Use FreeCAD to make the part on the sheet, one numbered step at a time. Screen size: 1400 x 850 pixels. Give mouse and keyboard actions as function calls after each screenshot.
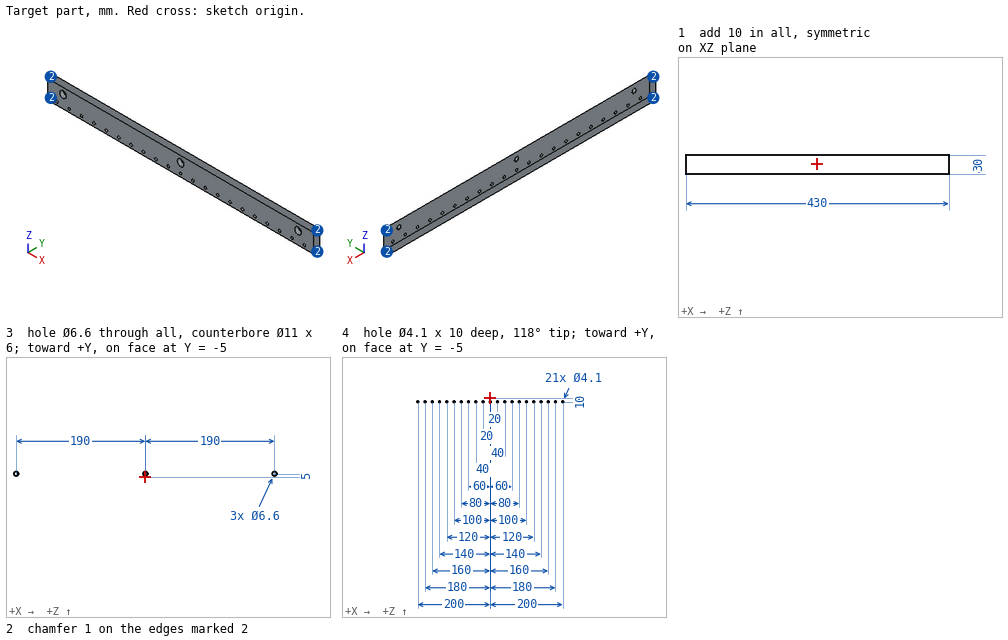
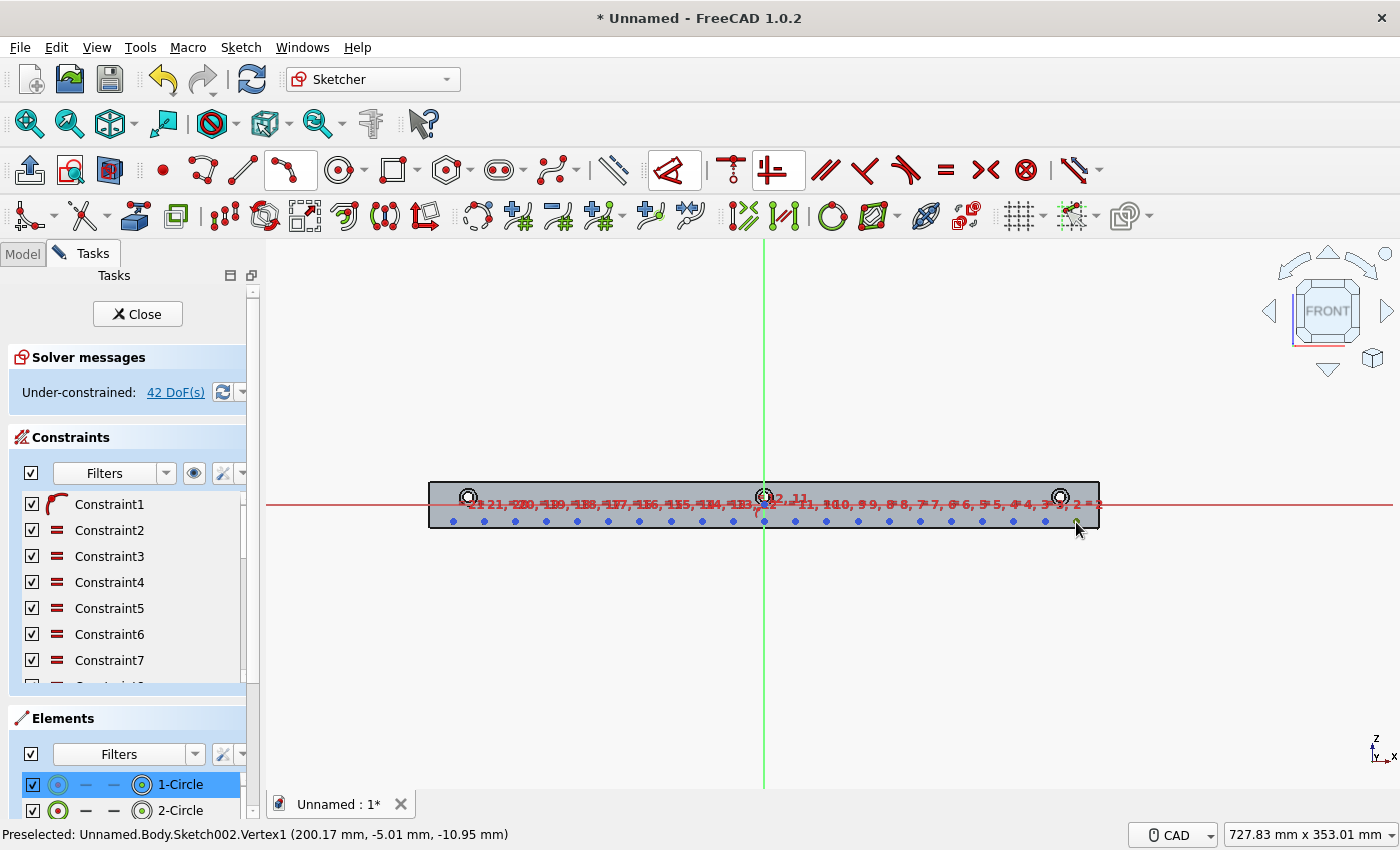
click(1045, 522)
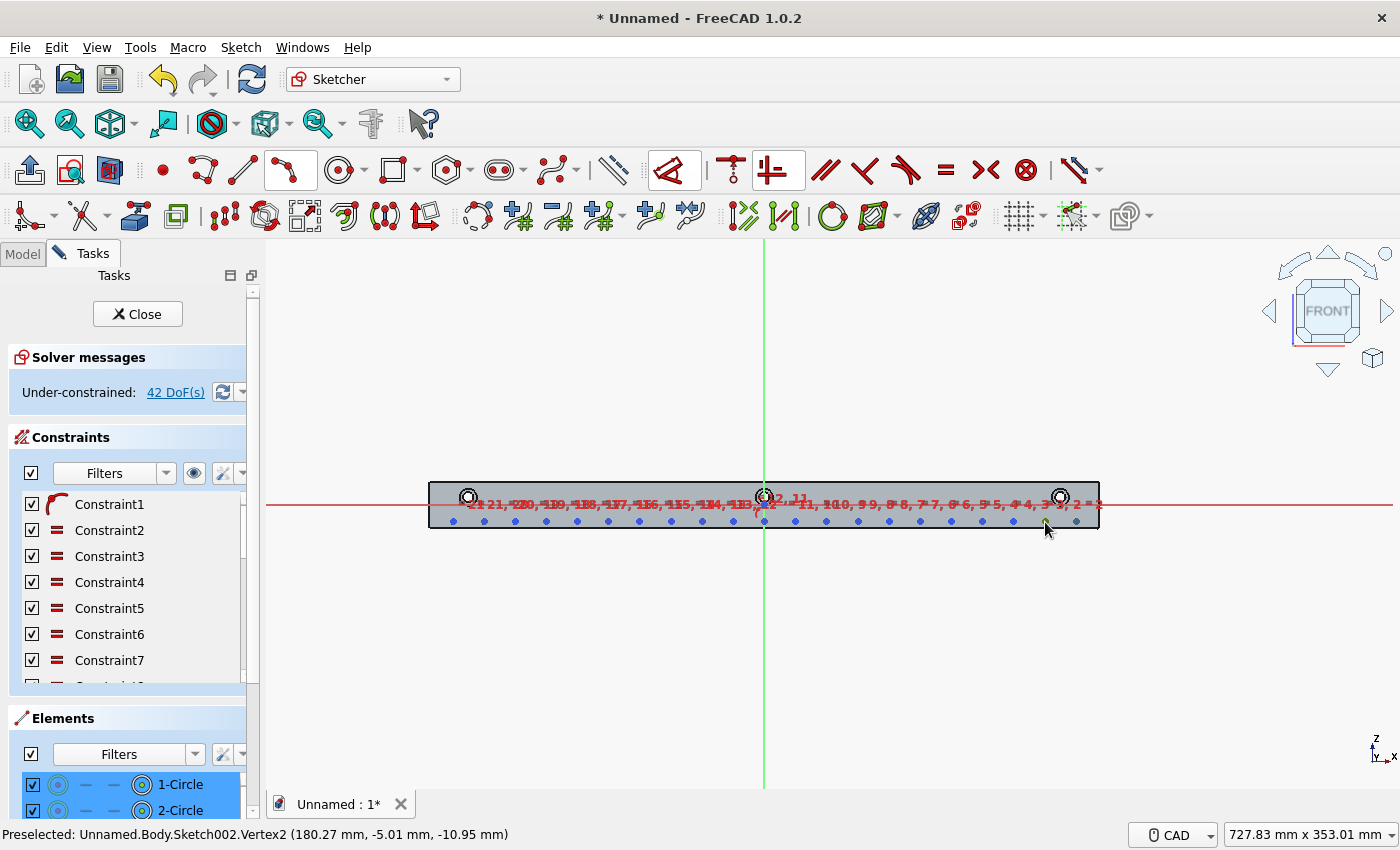
click(800, 170)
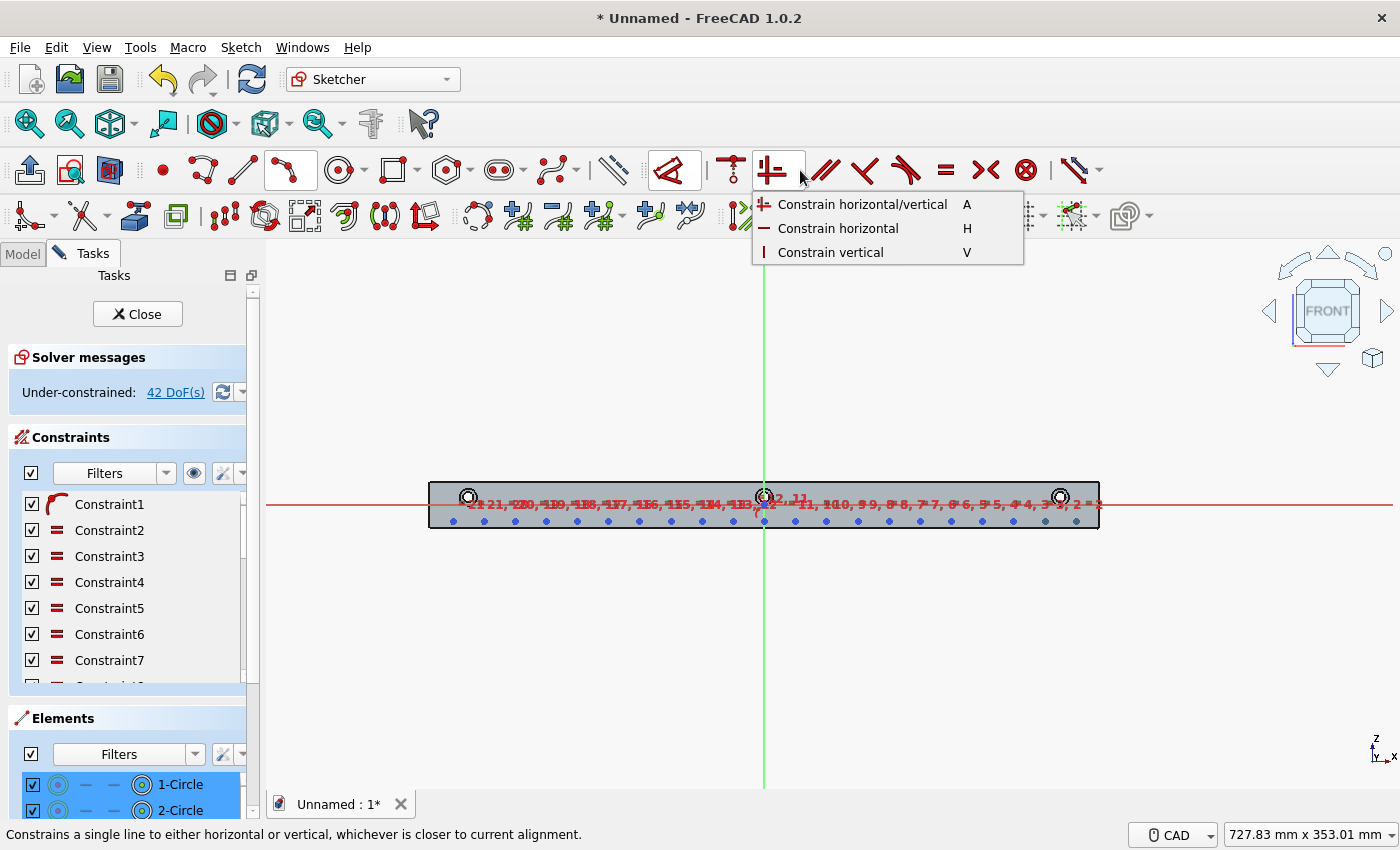
click(888, 228)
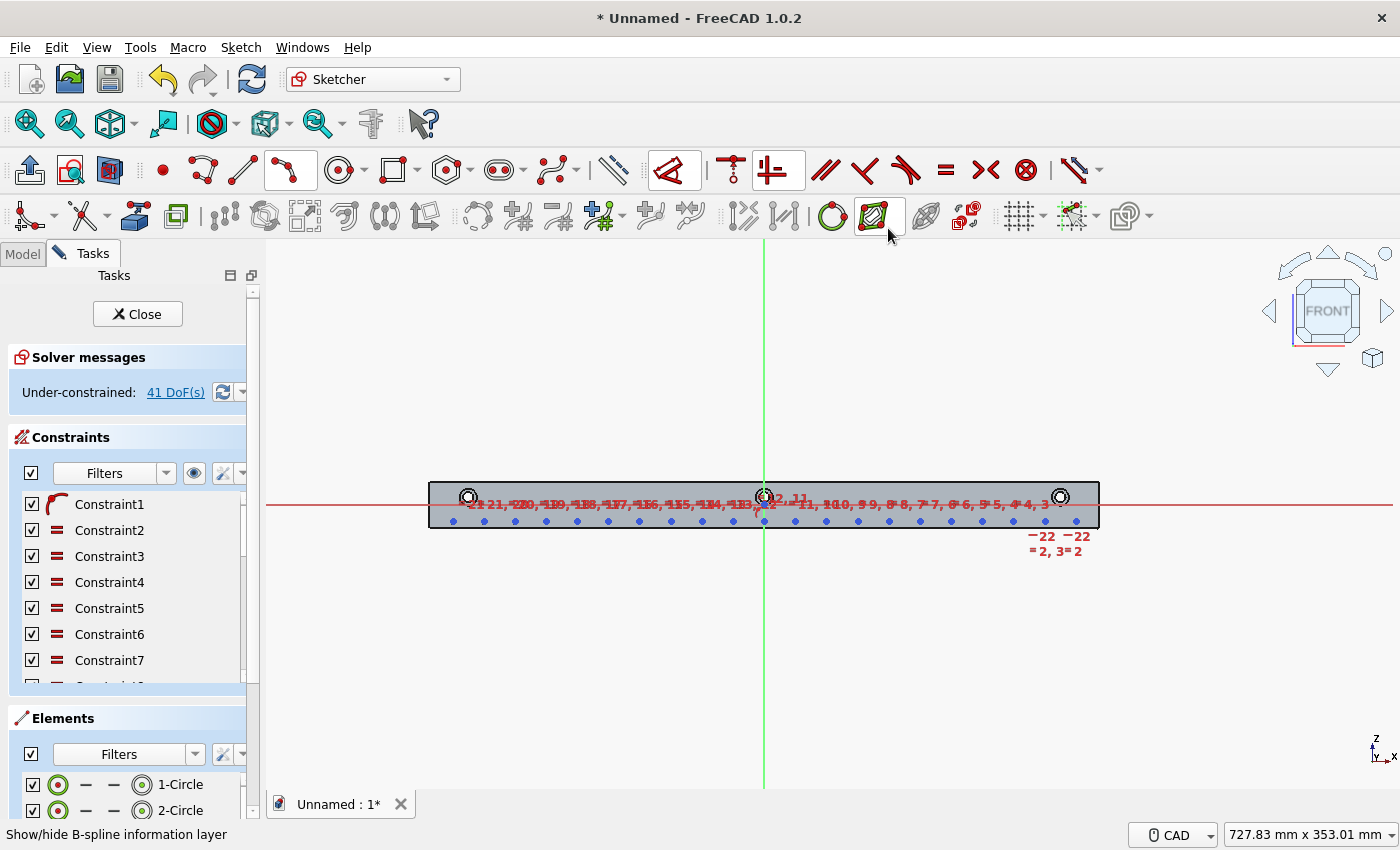
click(1045, 522)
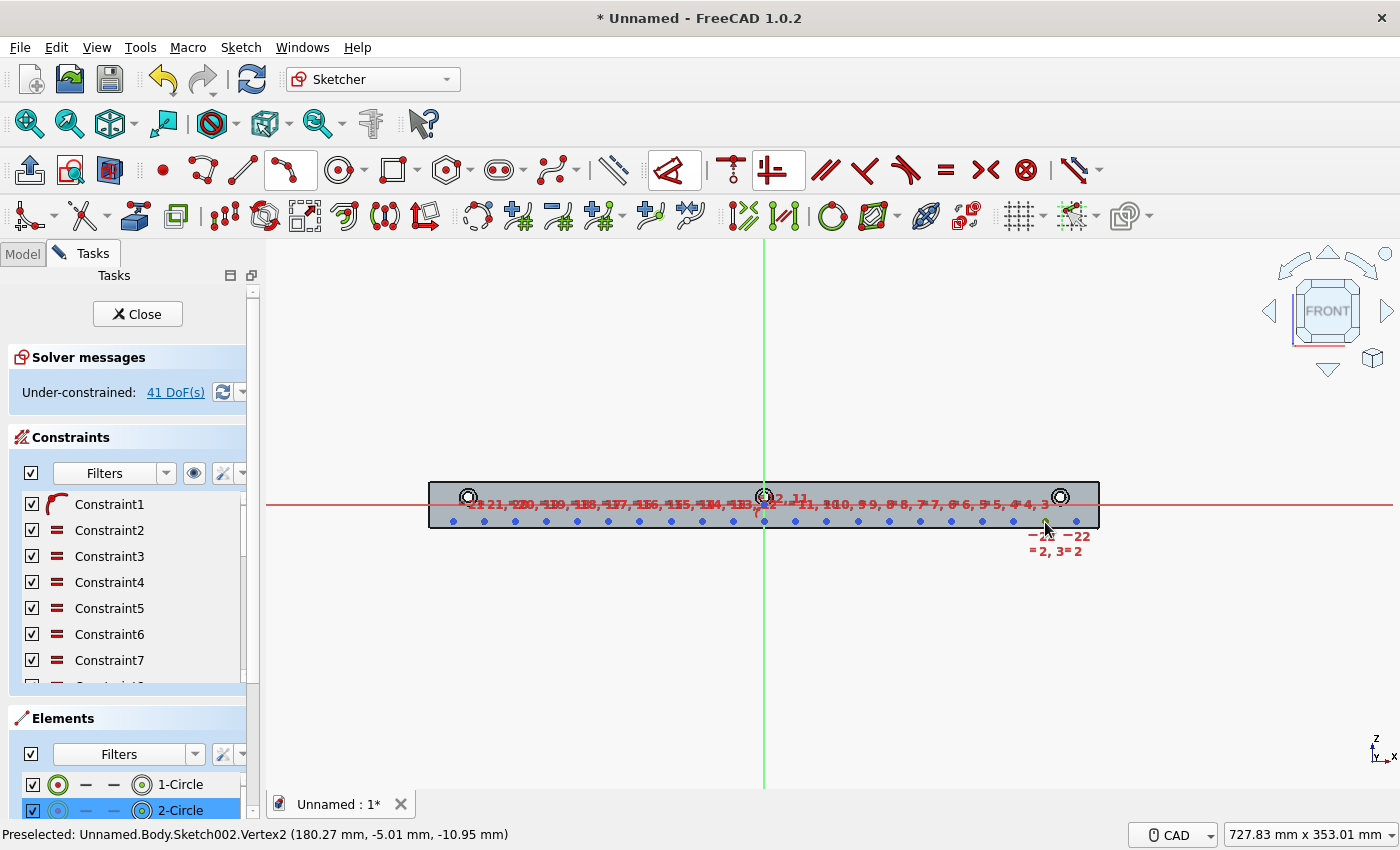
click(1013, 522)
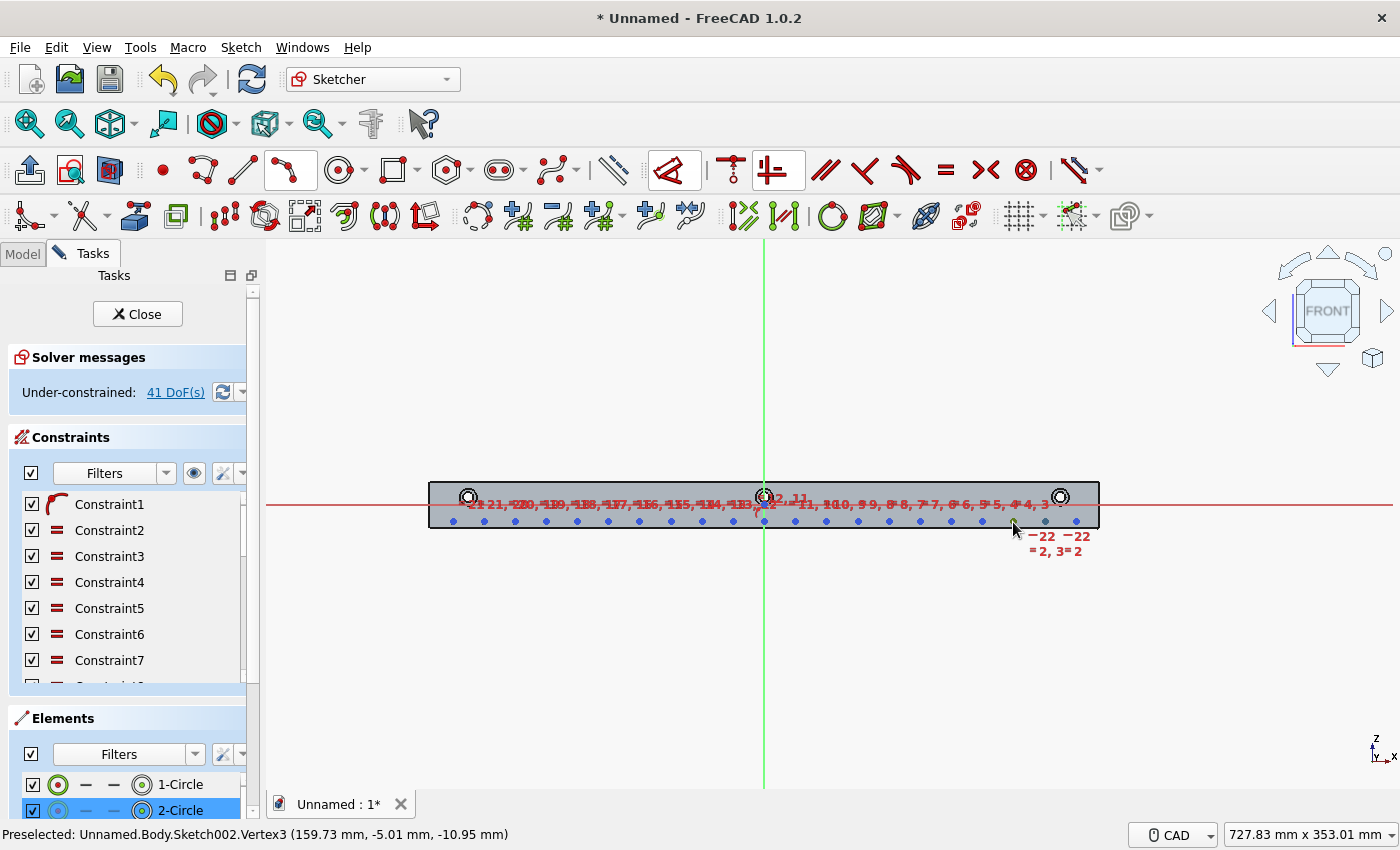
click(800, 170)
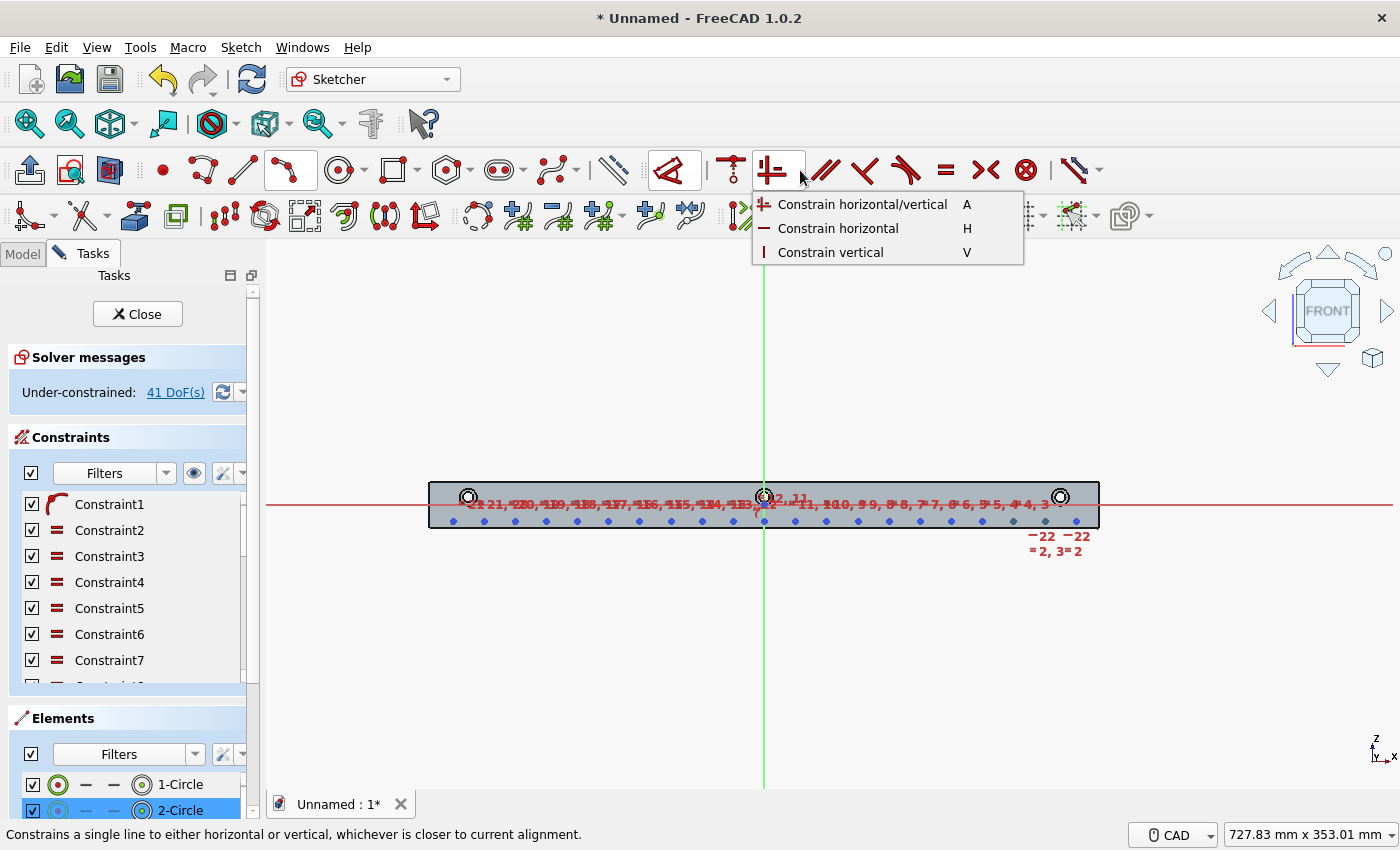
click(888, 228)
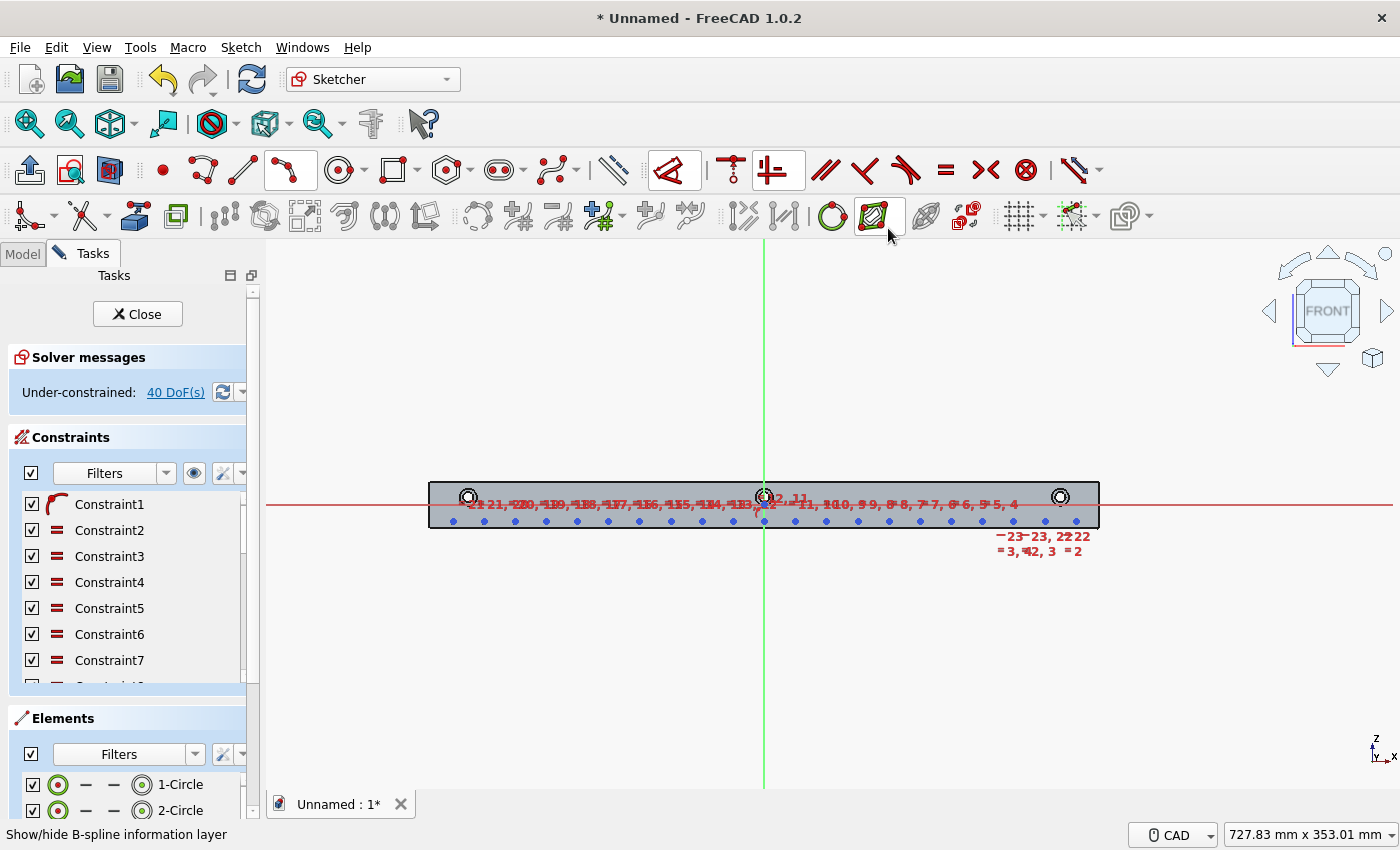
click(1013, 522)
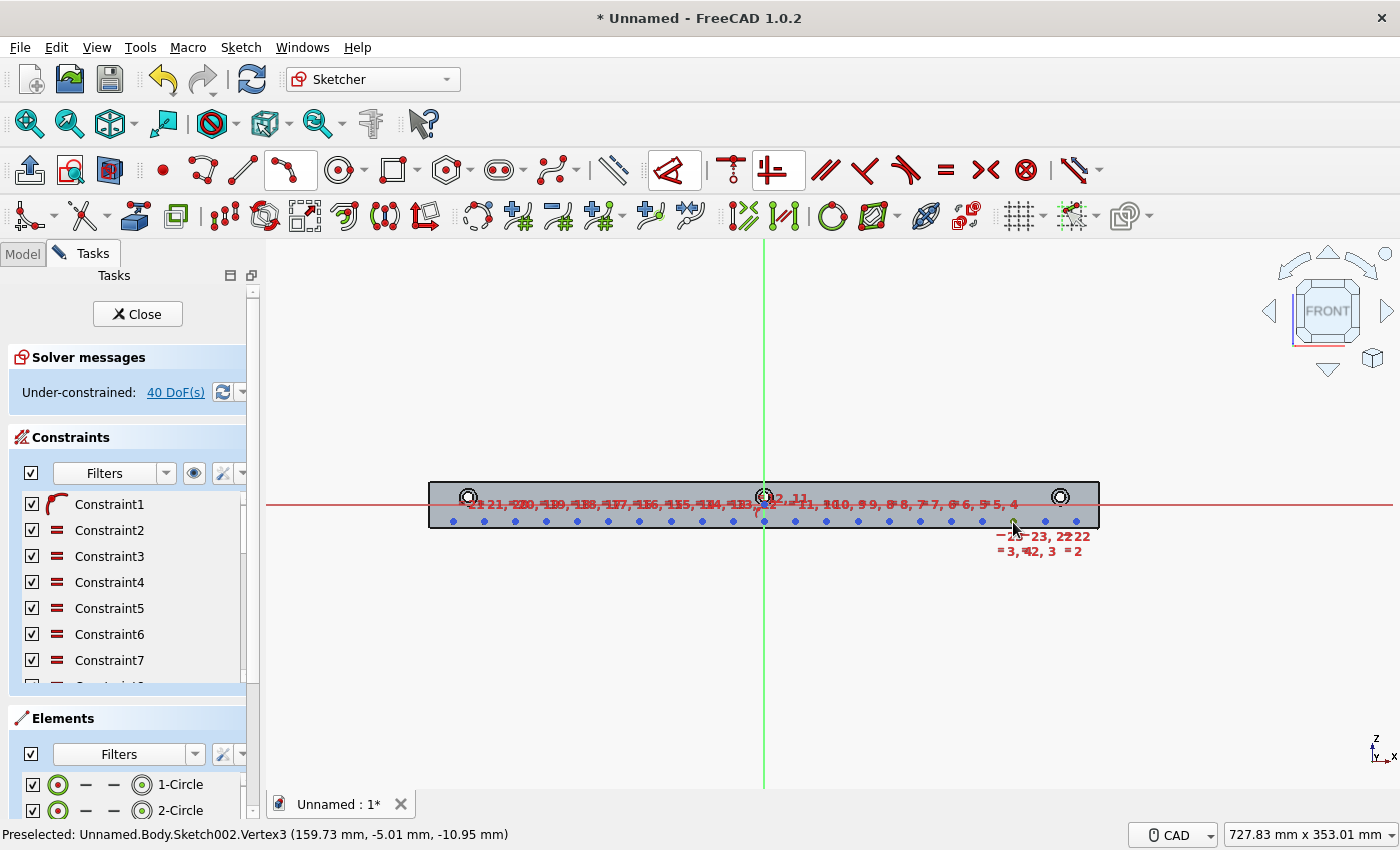
click(982, 522)